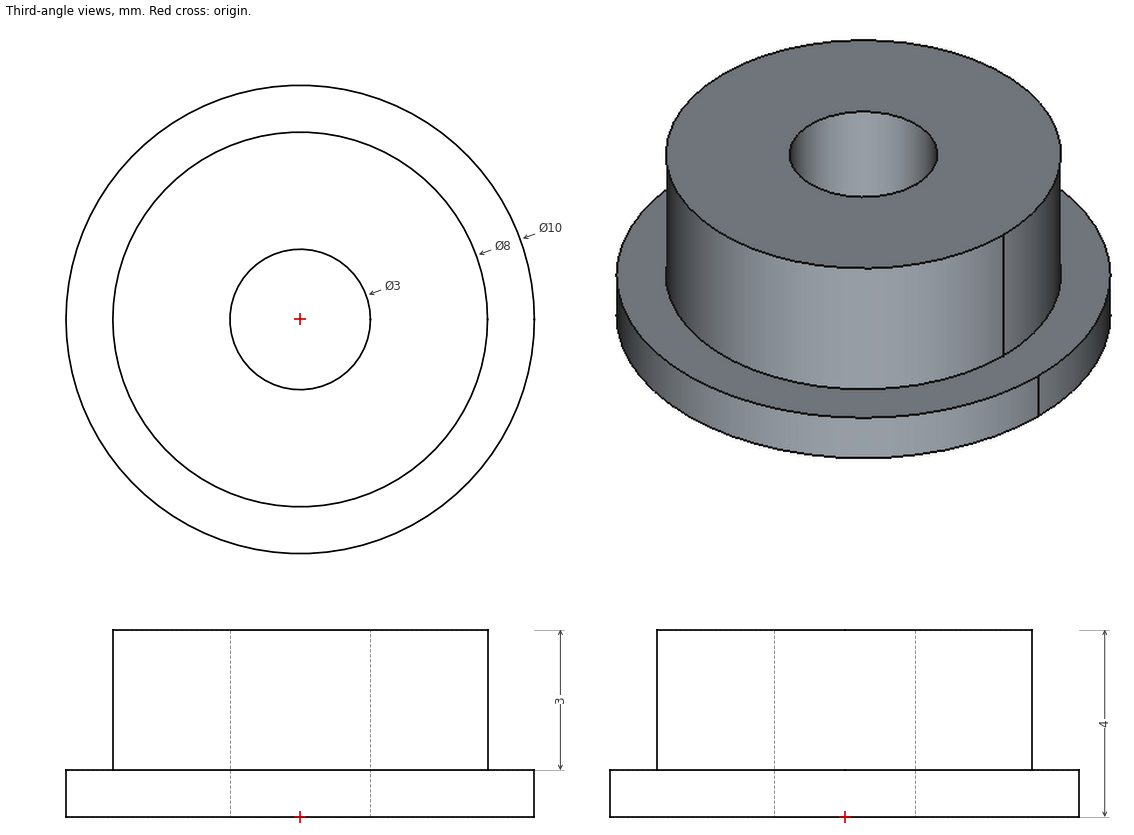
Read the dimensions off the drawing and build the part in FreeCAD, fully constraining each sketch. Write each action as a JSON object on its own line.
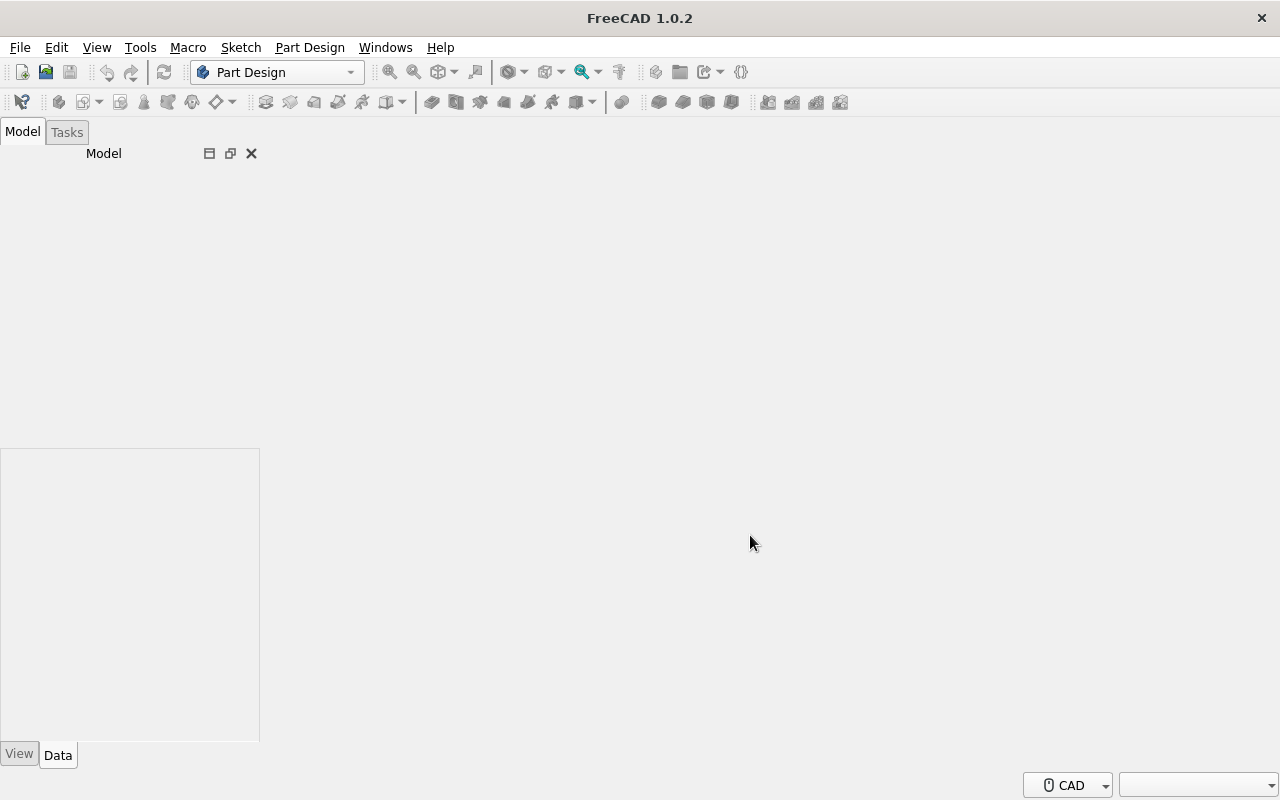
{"action": "left_click", "coordinate": [22, 72]}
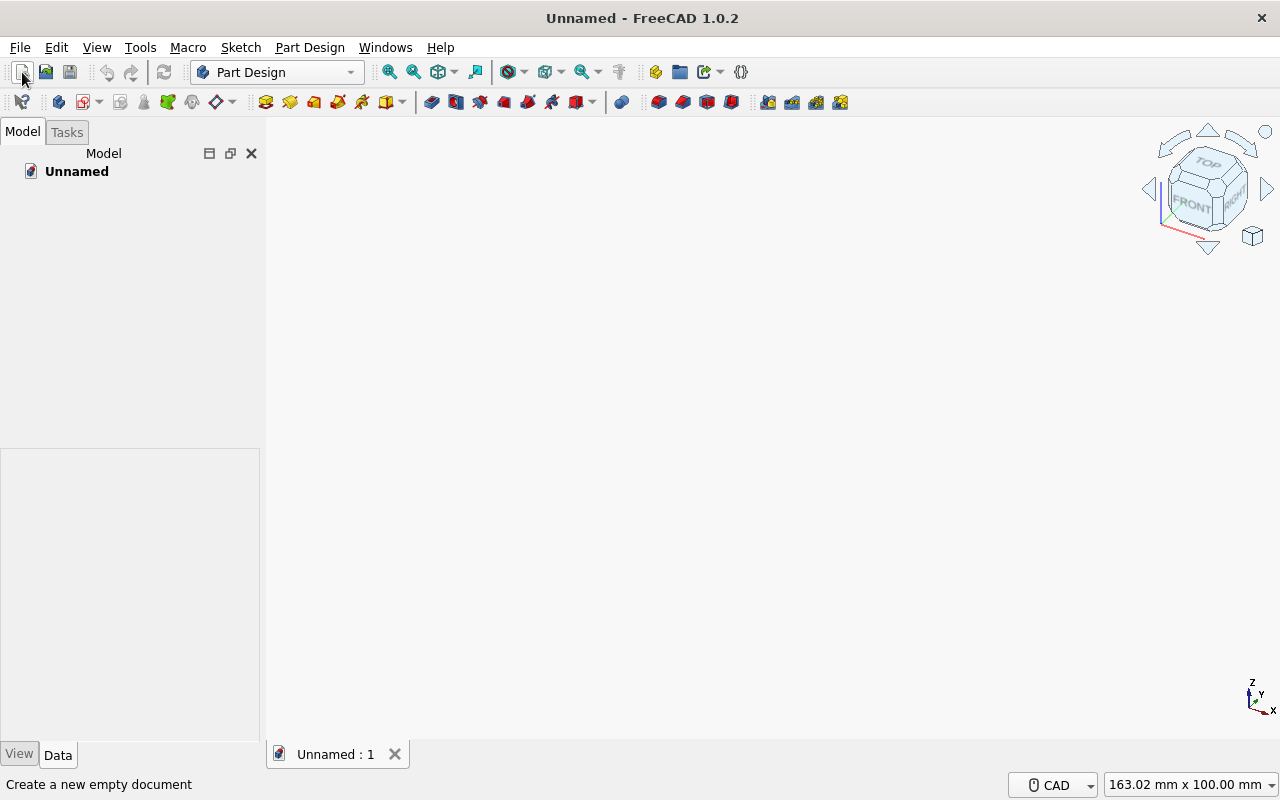
{"action": "left_click", "coordinate": [84, 102]}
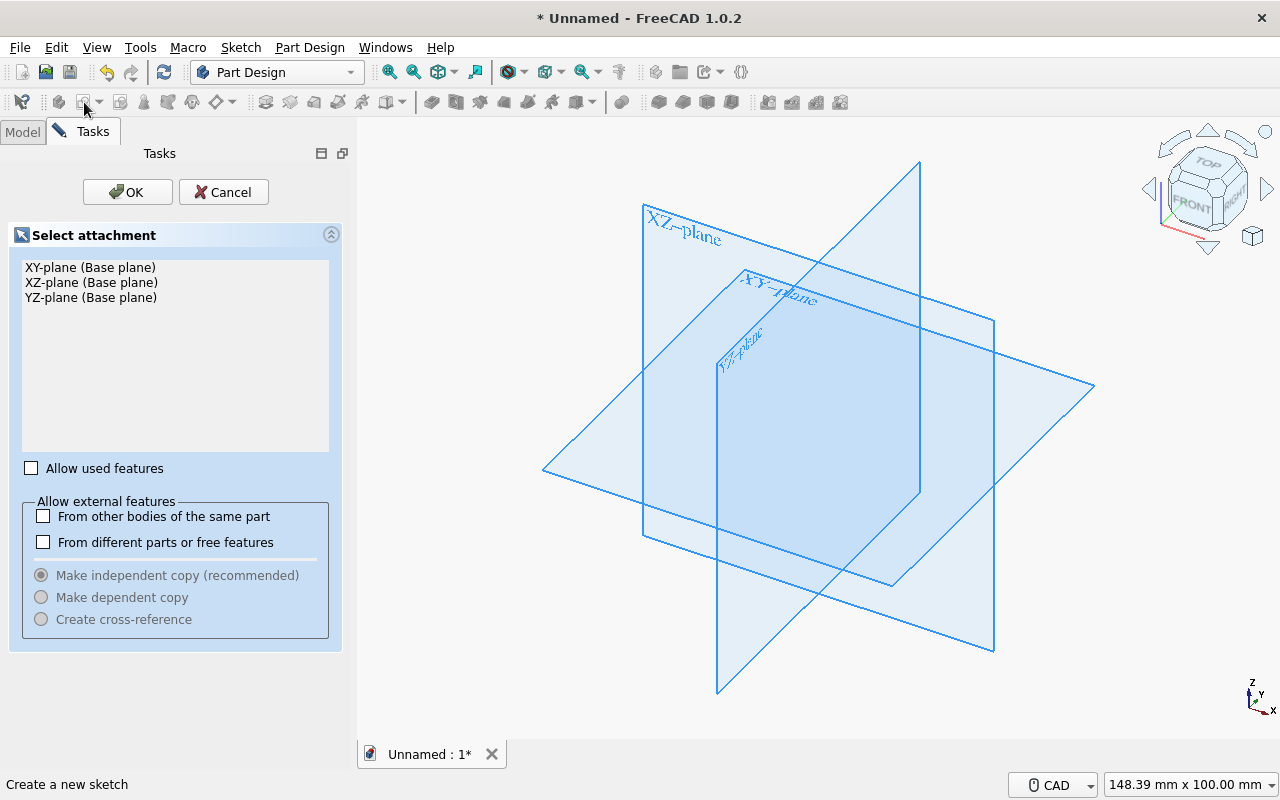
{"action": "left_click", "coordinate": [82, 268]}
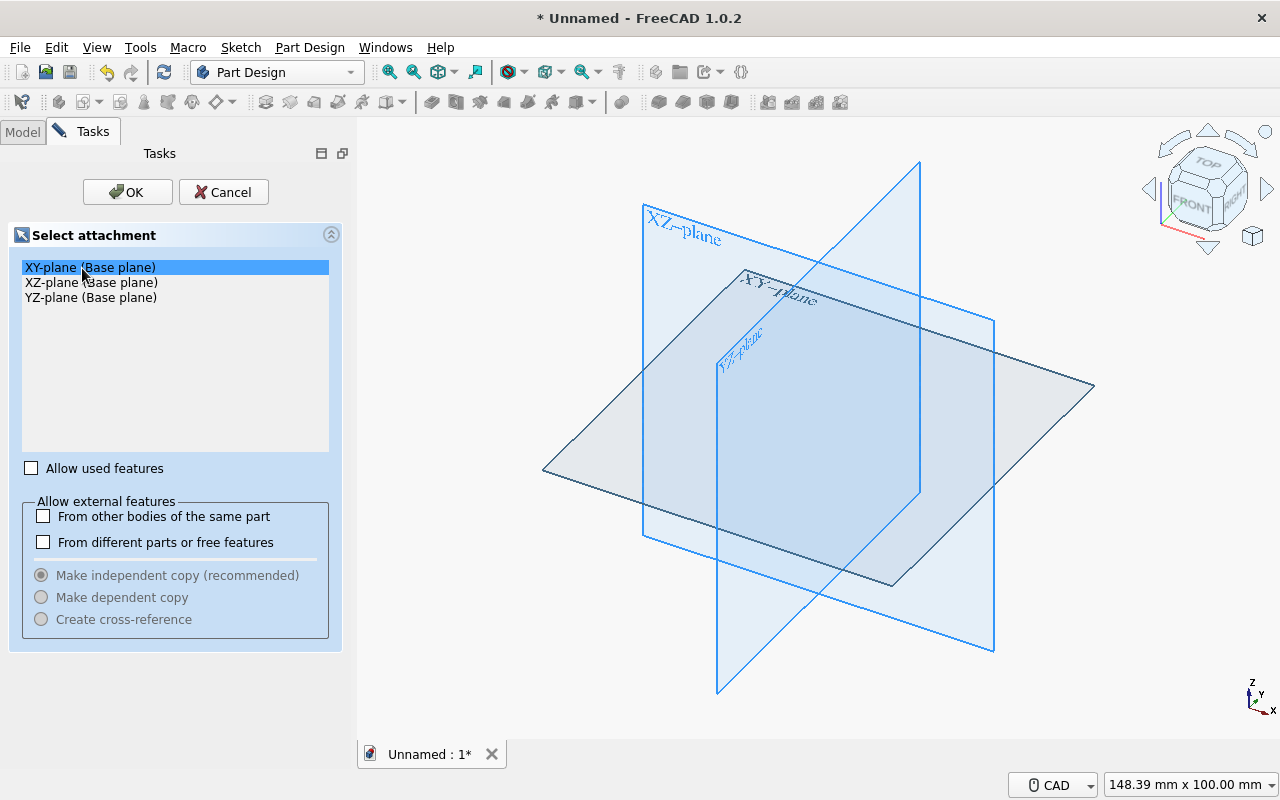
{"action": "left_click", "coordinate": [128, 192]}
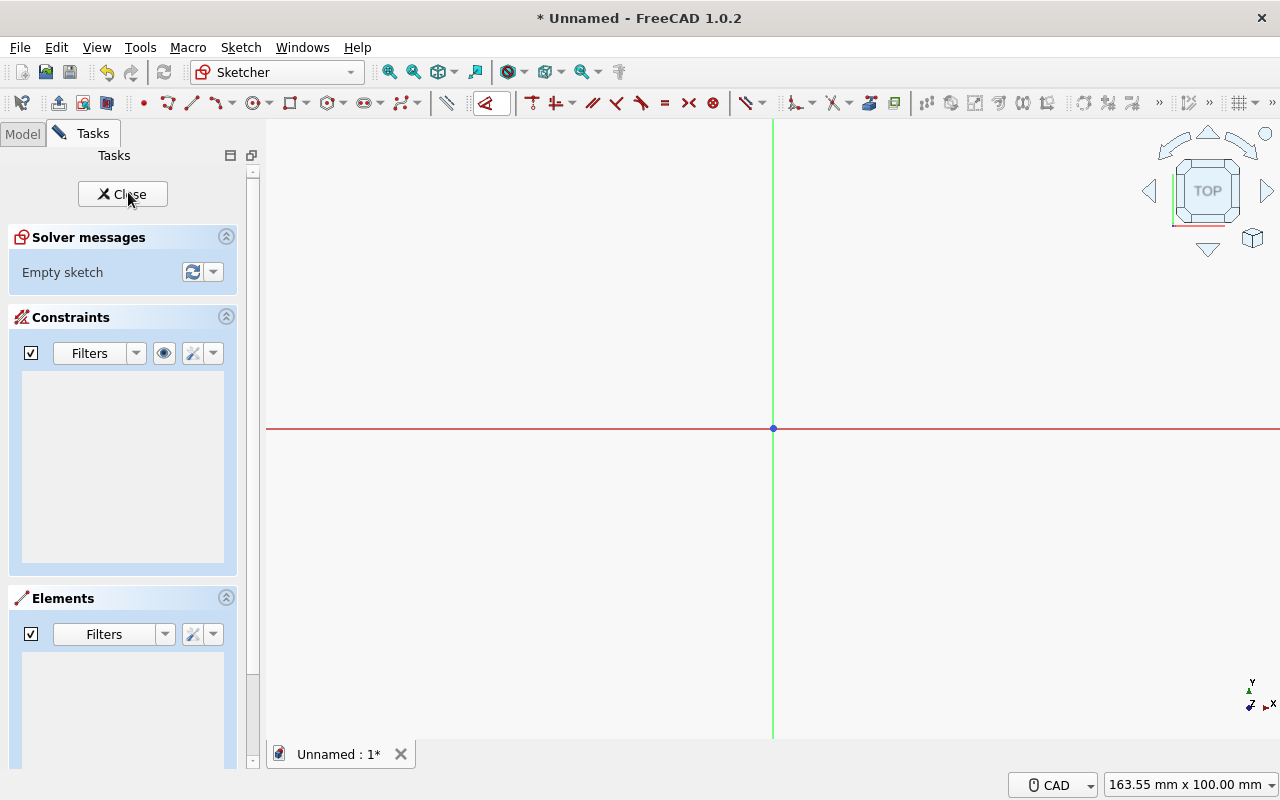
{"action": "scroll", "coordinate": [787, 429], "scroll_direction": "up", "scroll_amount": 9}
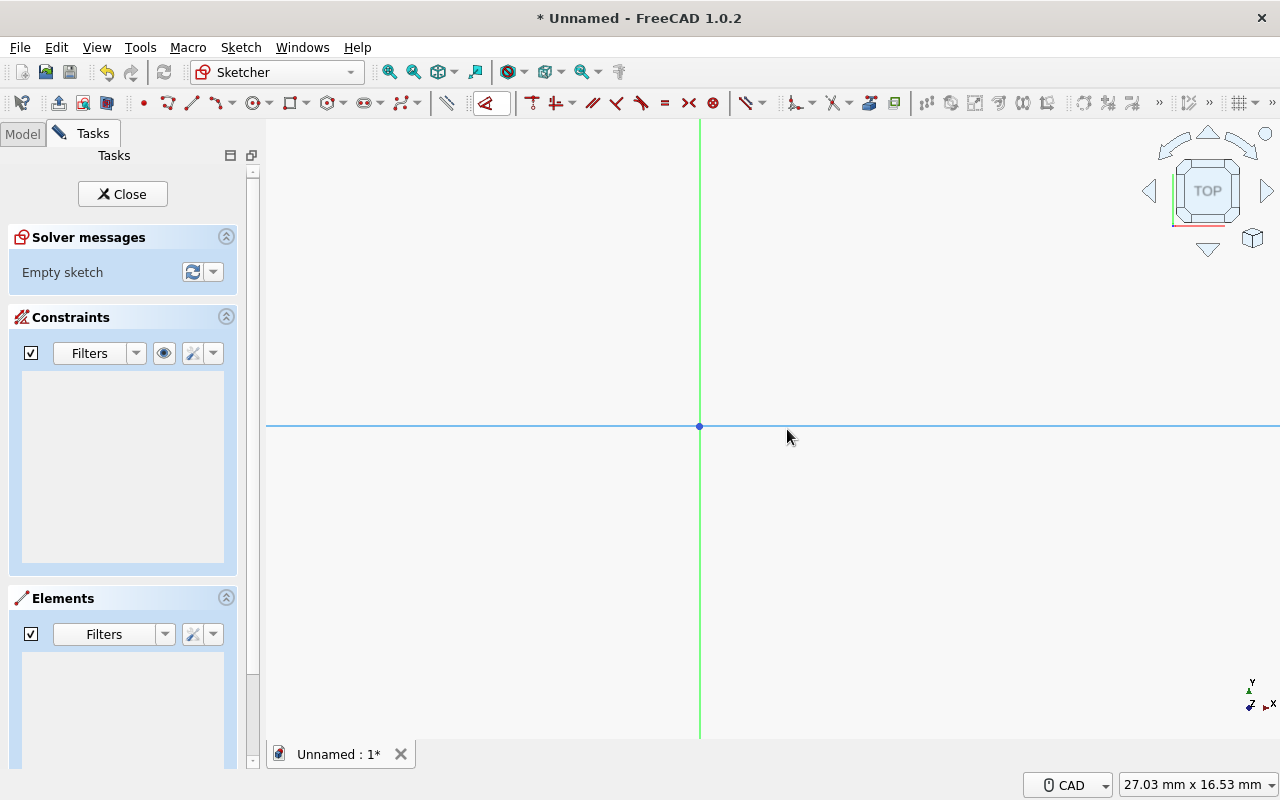
{"action": "key", "text": "g c"}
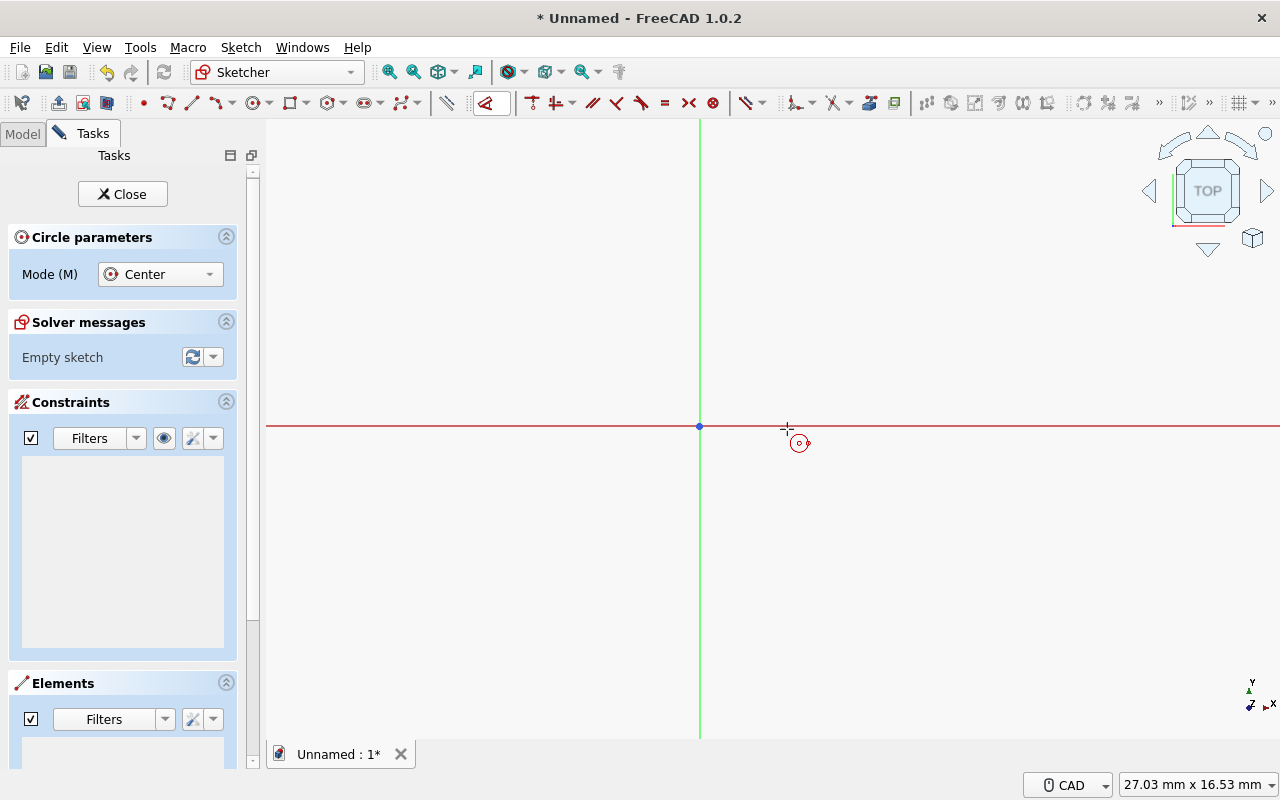
{"action": "left_click", "coordinate": [700, 426]}
{"action": "left_click", "coordinate": [832, 294]}
{"action": "key", "text": "Escape"}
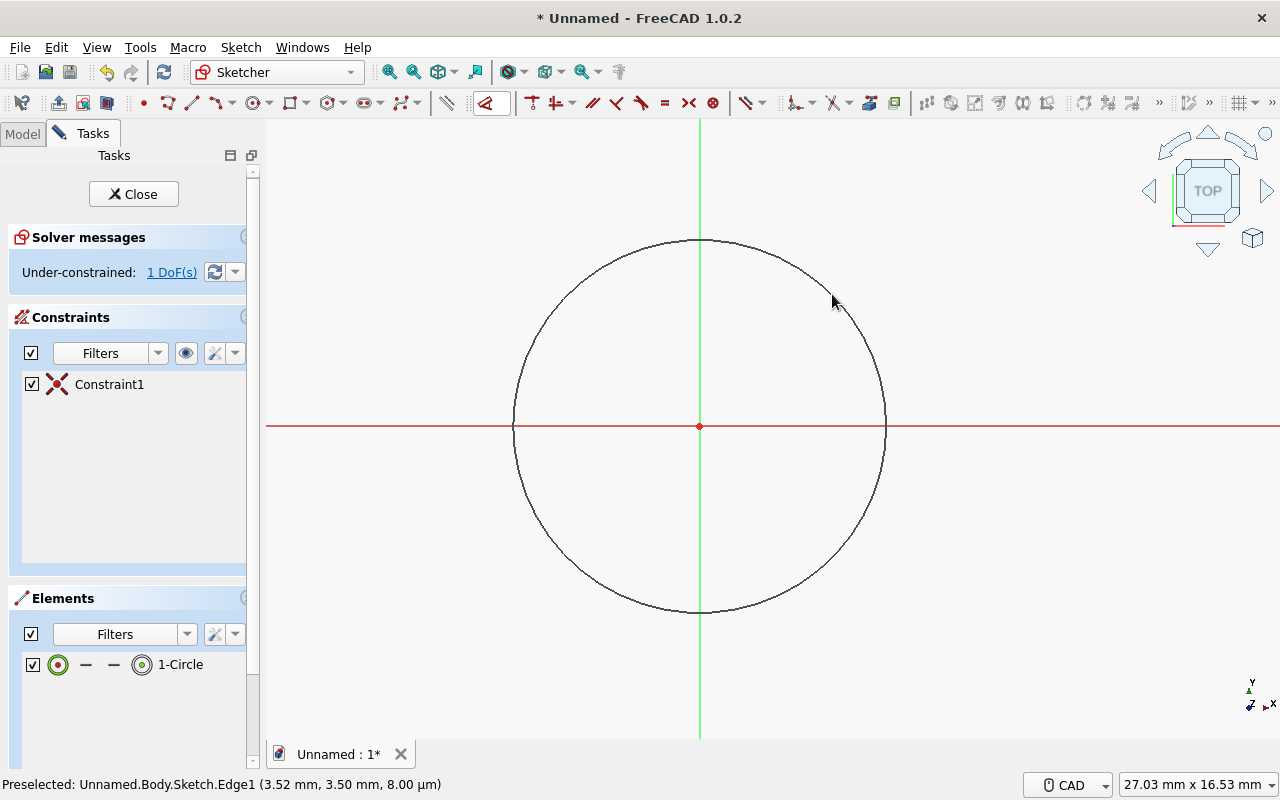
{"action": "left_click", "coordinate": [831, 294]}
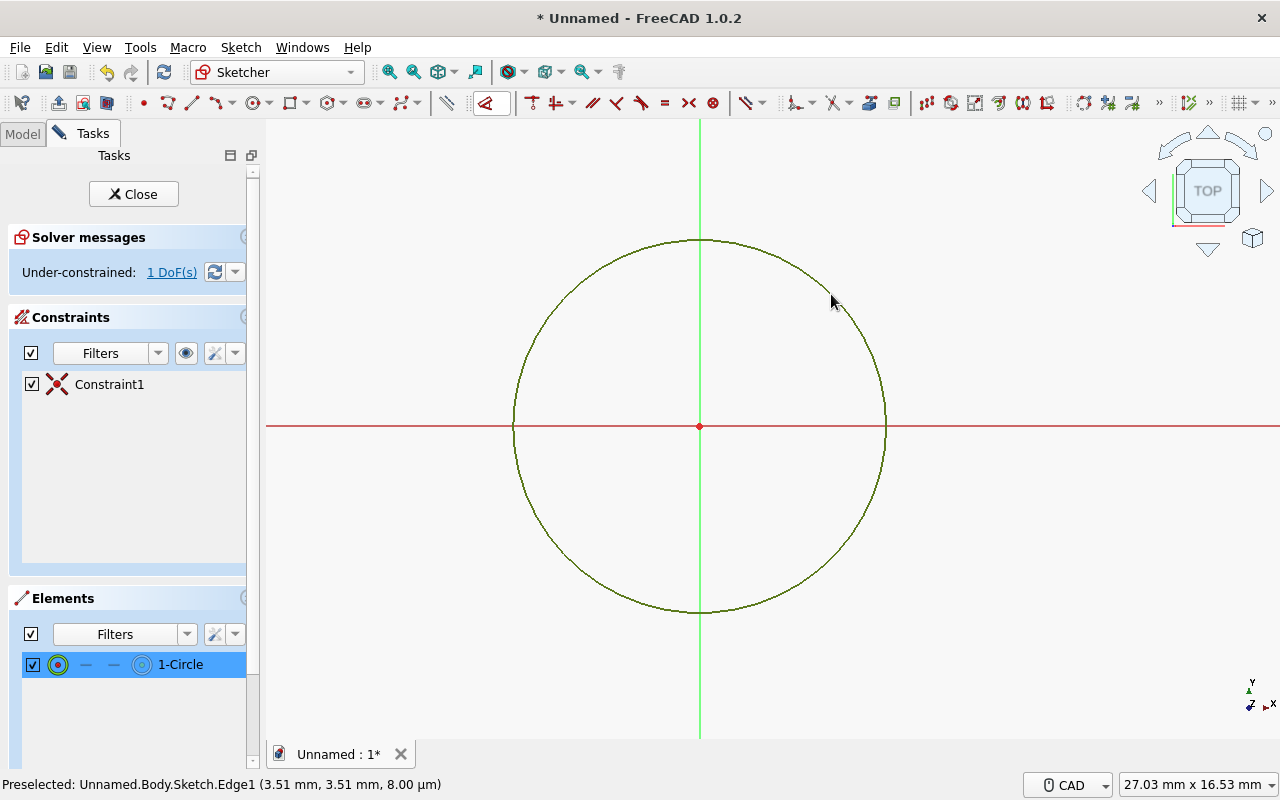
{"action": "key", "text": "k o"}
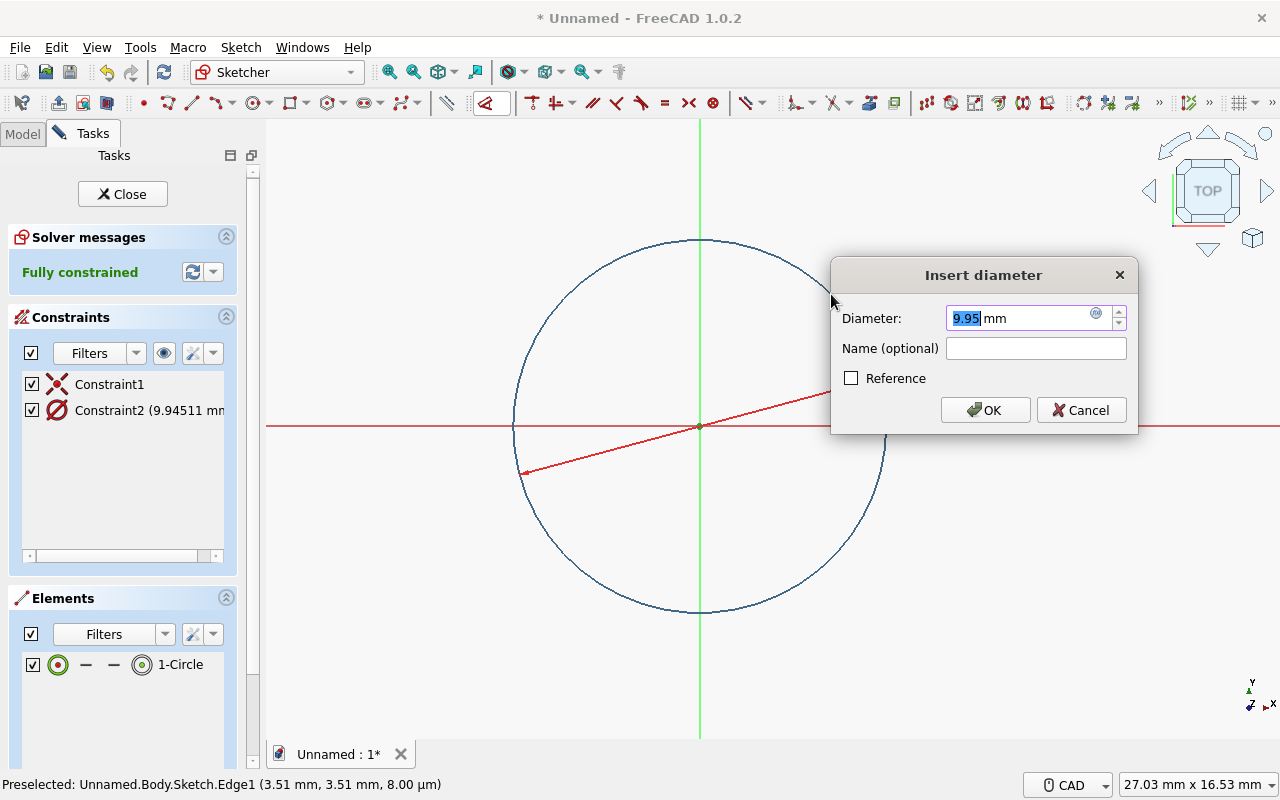
{"action": "type", "text": "10"}
{"action": "key", "text": "Return"}